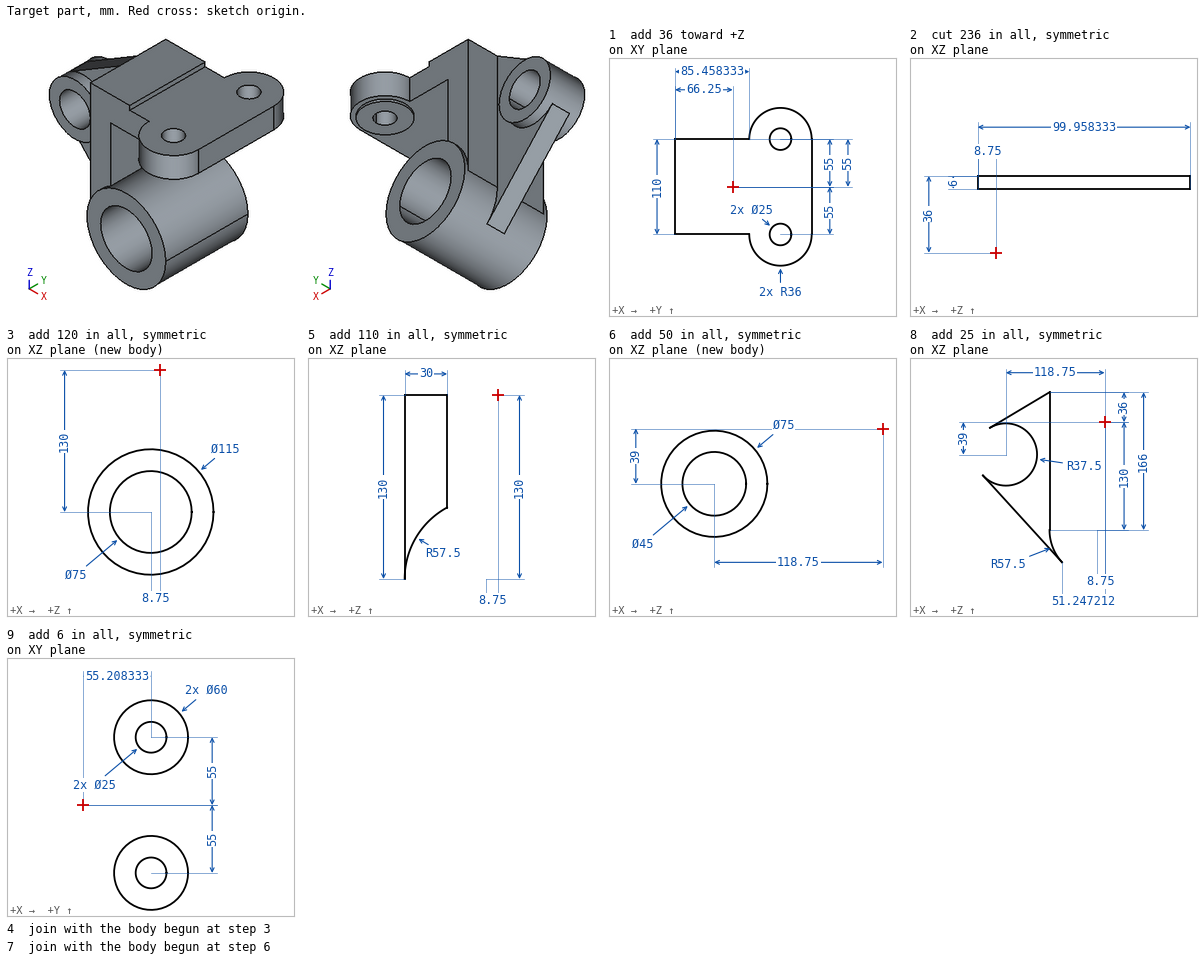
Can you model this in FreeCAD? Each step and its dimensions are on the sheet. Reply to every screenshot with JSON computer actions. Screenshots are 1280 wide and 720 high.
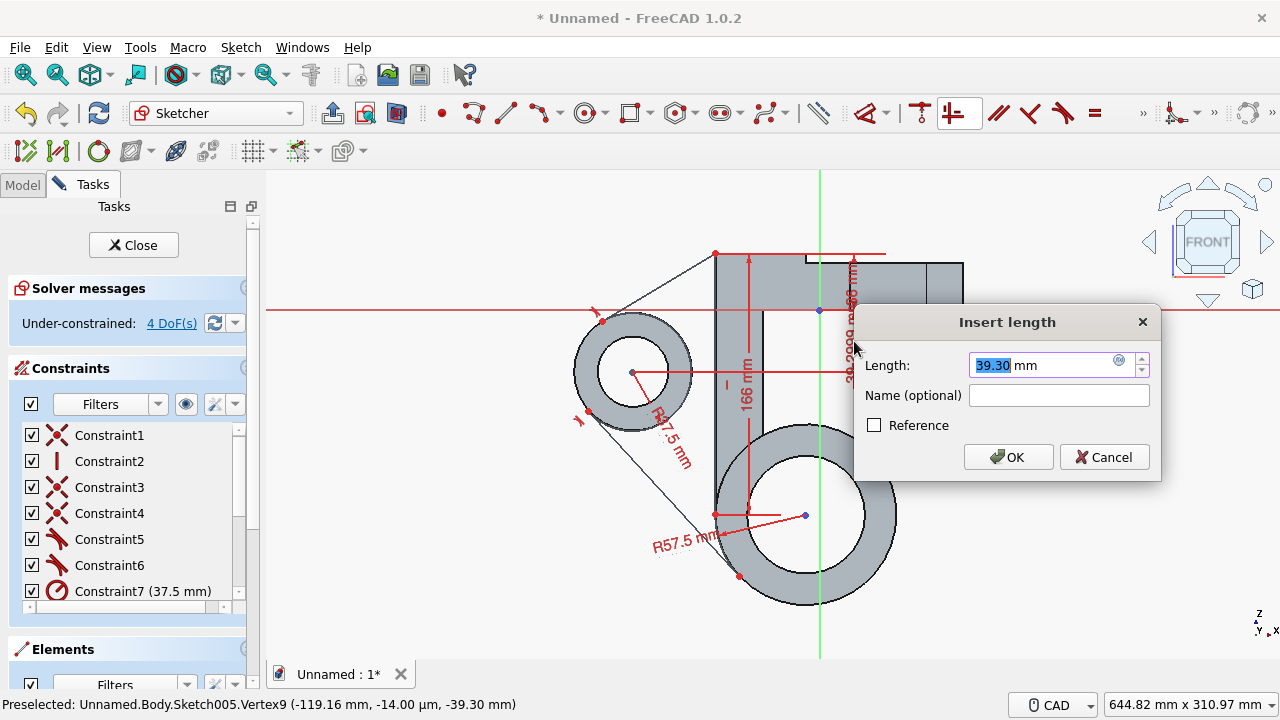
{"action": "type", "text": "39"}
{"action": "key", "text": "Return"}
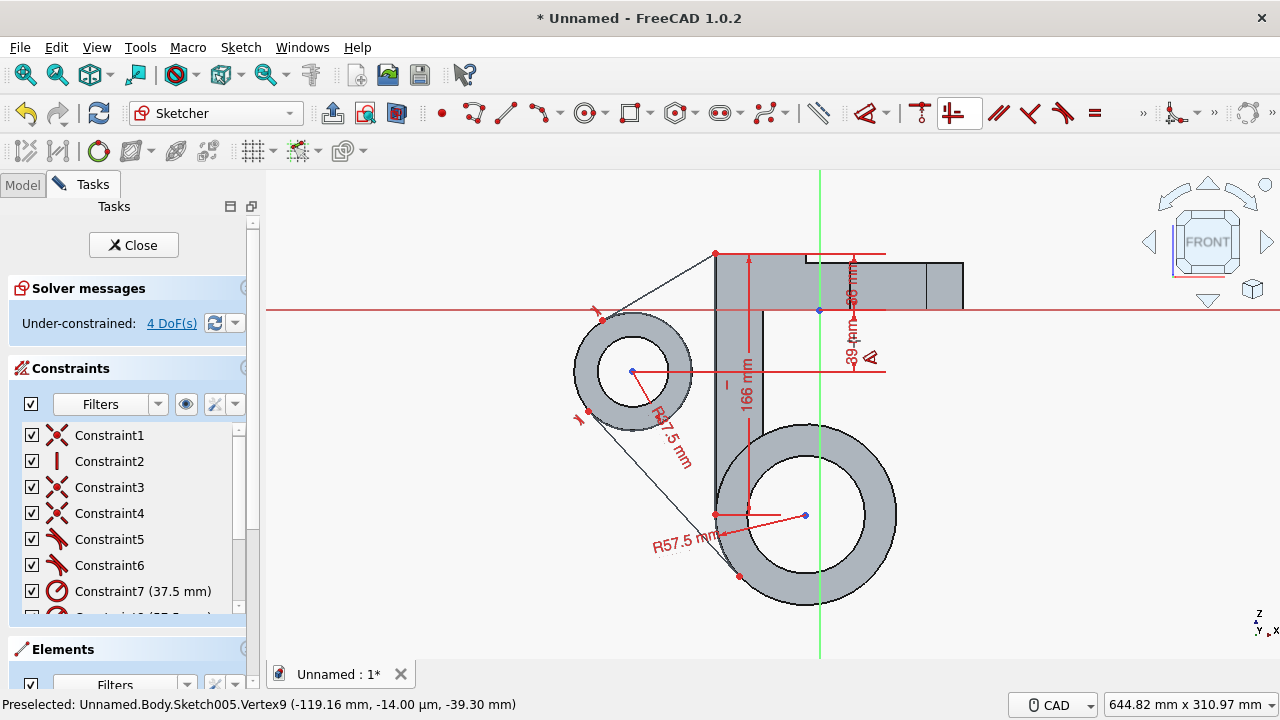
{"action": "left_click", "coordinate": [806, 515]}
{"action": "left_click", "coordinate": [854, 413]}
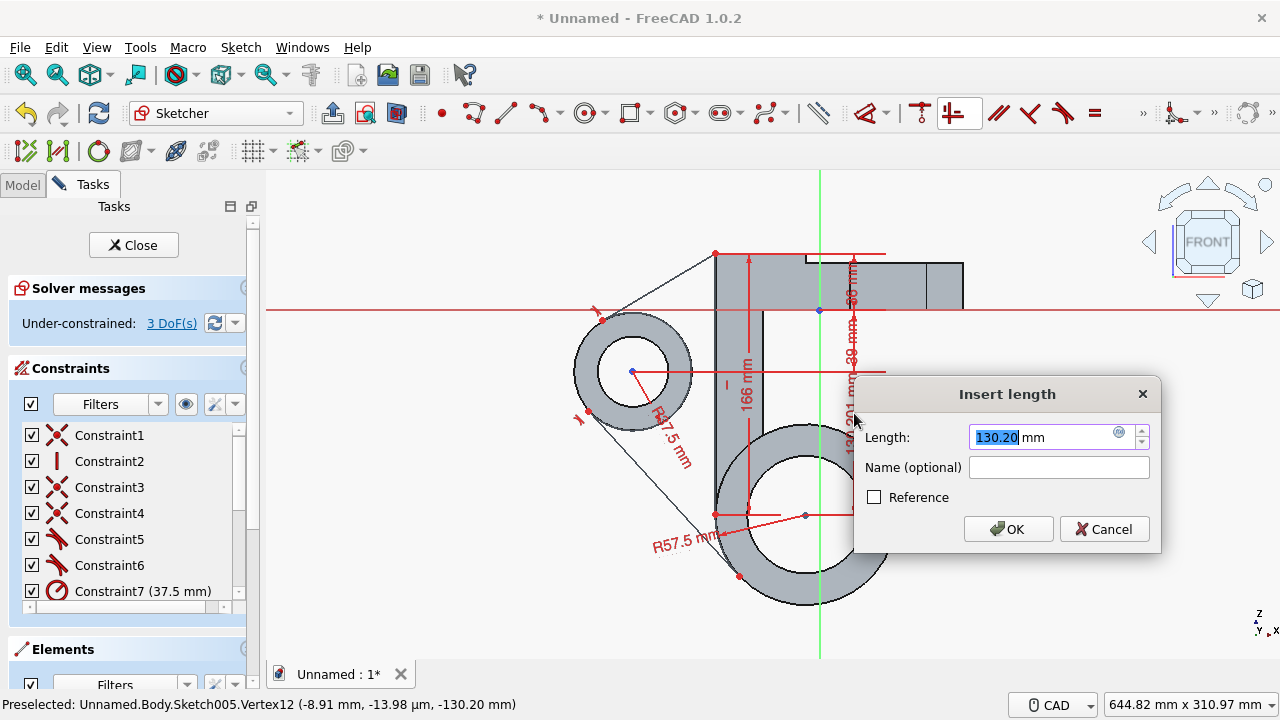
{"action": "type", "text": "130"}
{"action": "key", "text": "Return"}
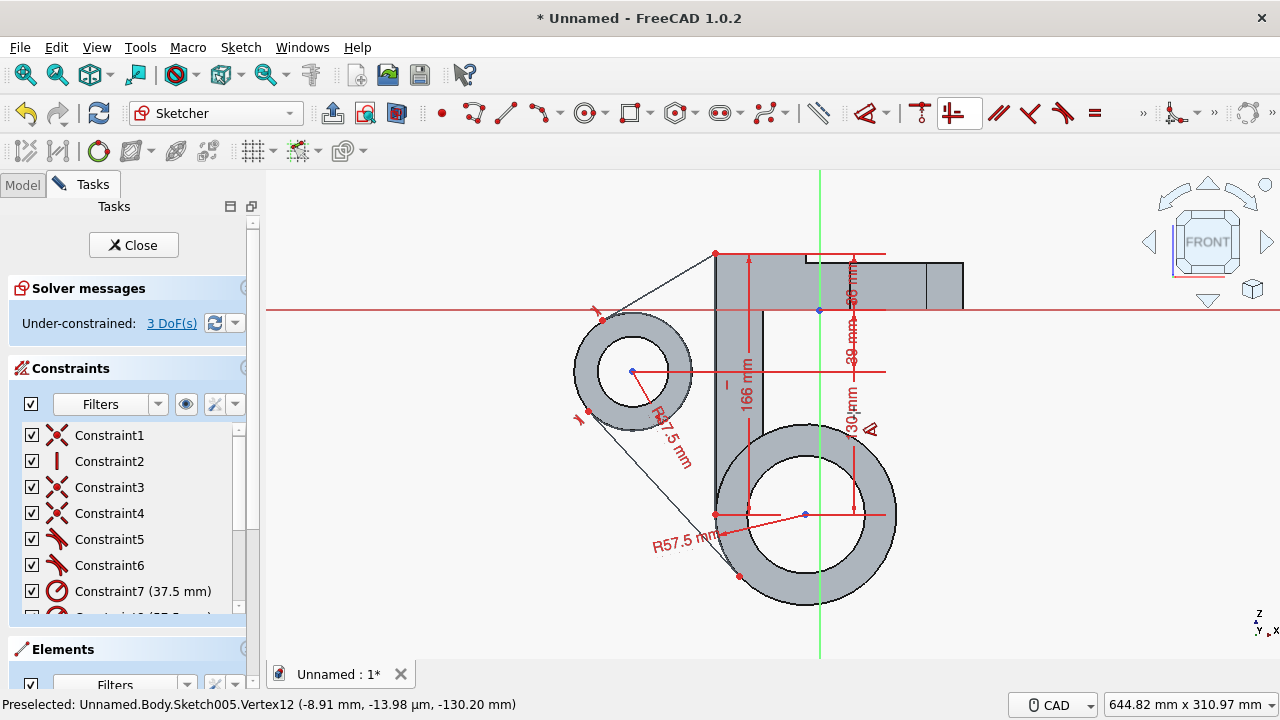
{"action": "scroll", "coordinate": [806, 515], "scroll_direction": "up", "scroll_amount": 6}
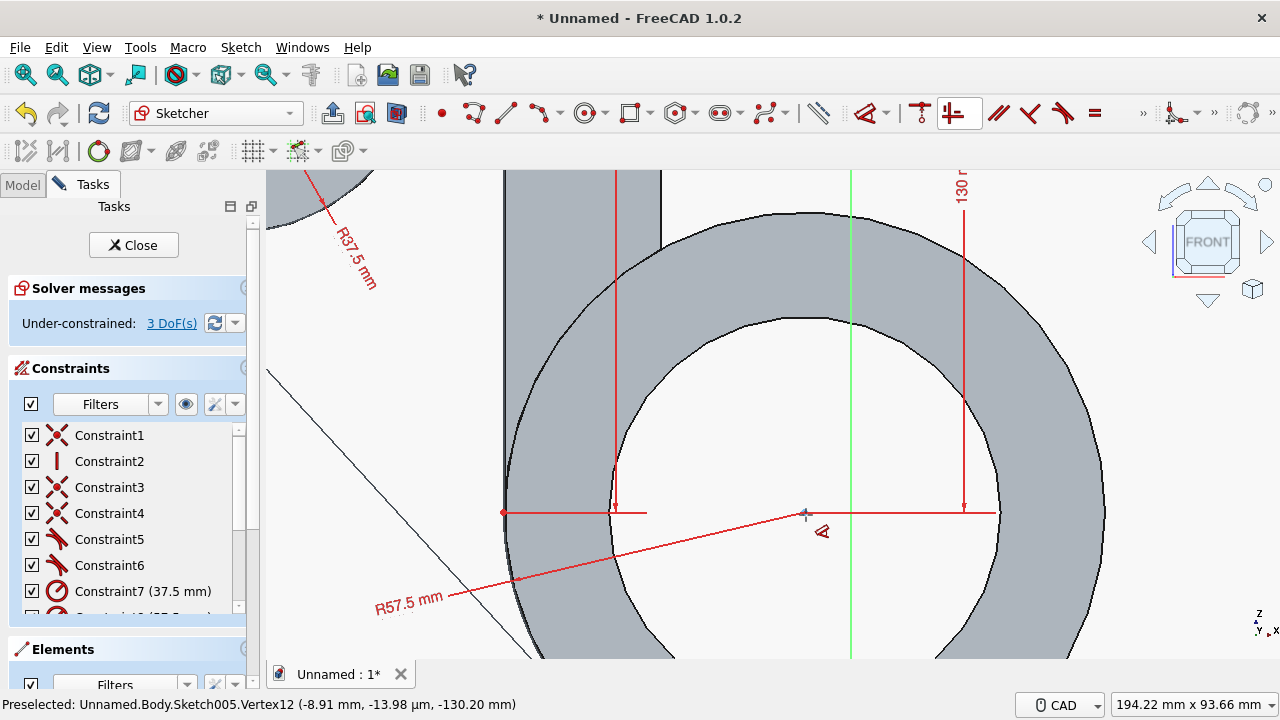
{"action": "left_click", "coordinate": [804, 513]}
{"action": "left_click", "coordinate": [827, 547]}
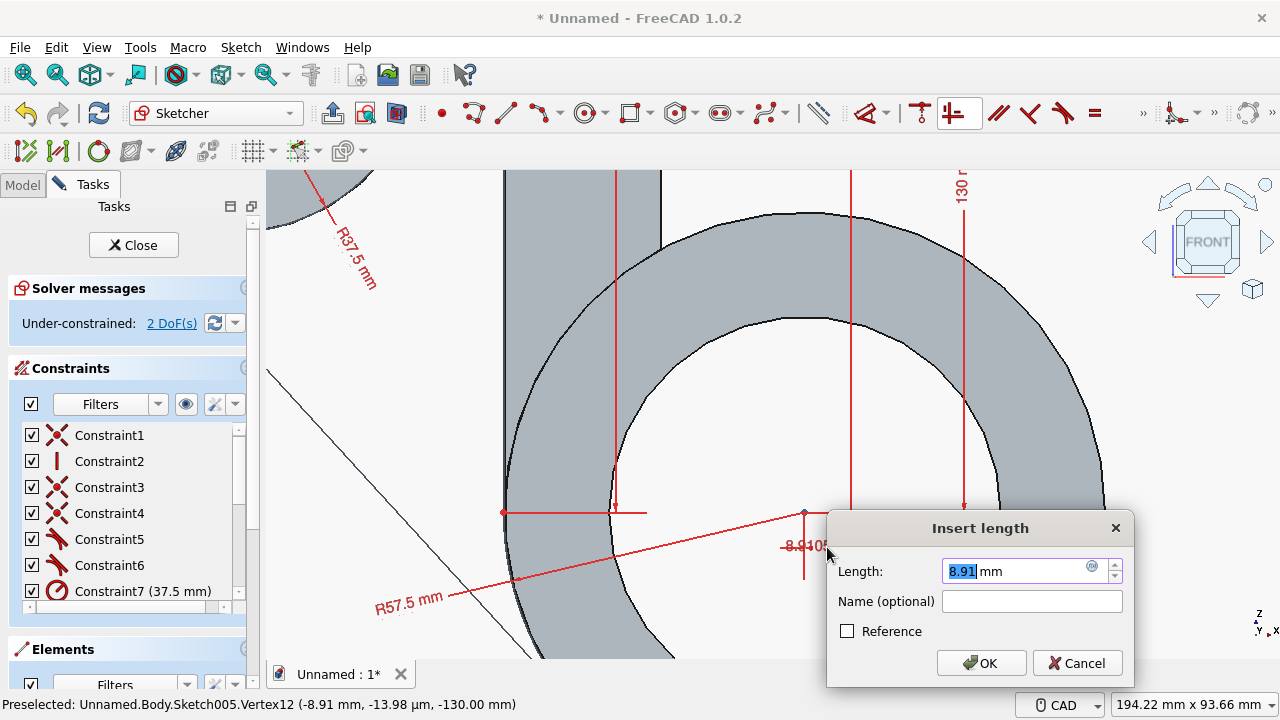
{"action": "type", "text": "8.75"}
{"action": "key", "text": "Return"}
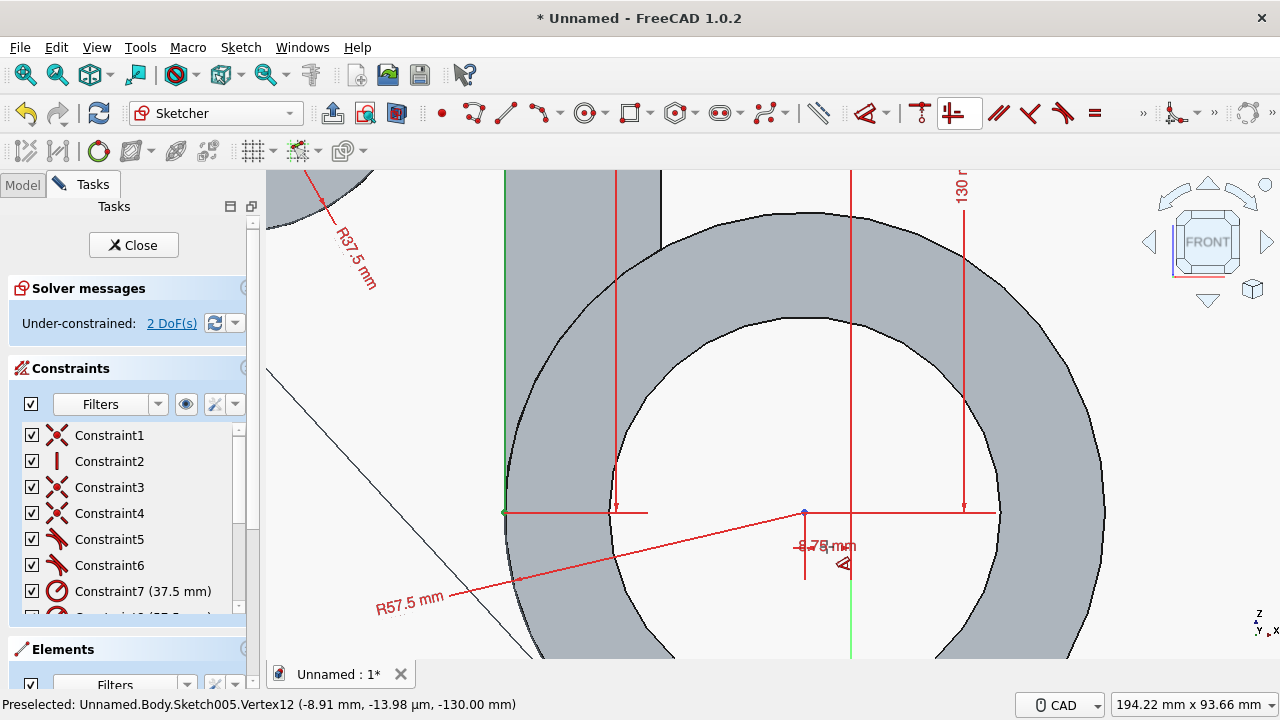
{"action": "scroll", "coordinate": [806, 515], "scroll_direction": "down", "scroll_amount": 6}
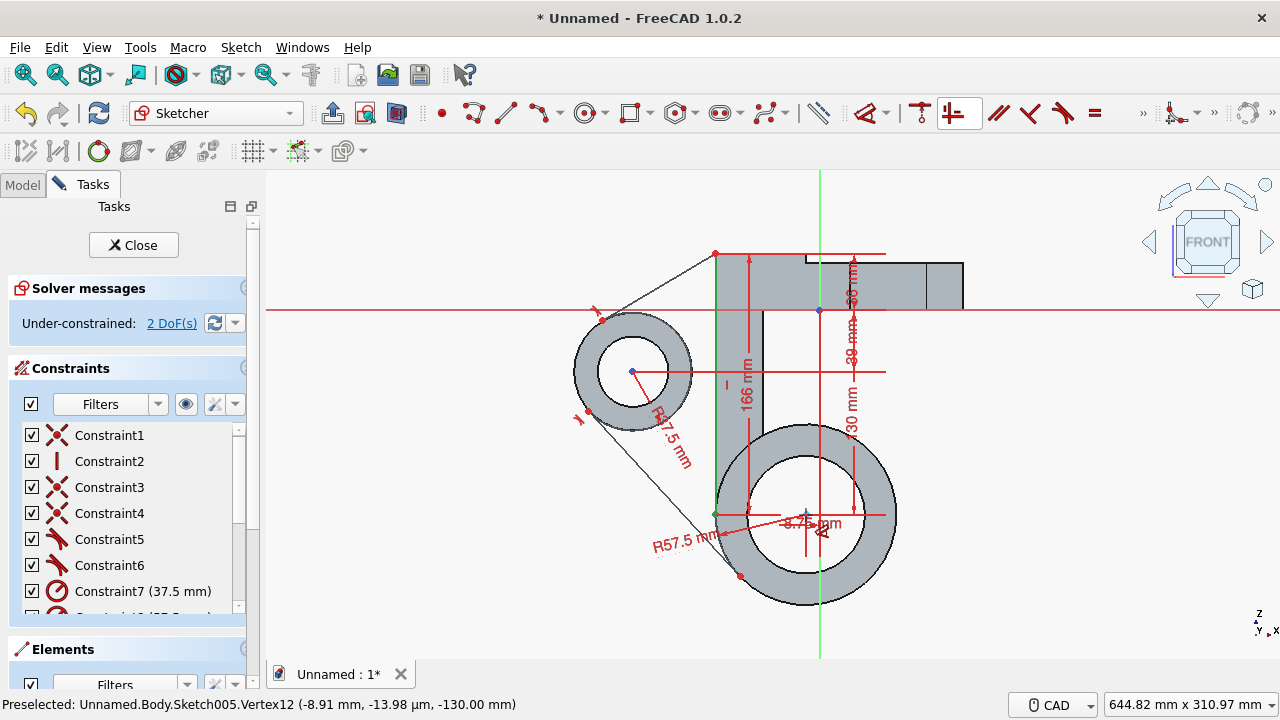
{"action": "left_click", "coordinate": [632, 372]}
{"action": "left_click", "coordinate": [769, 276]}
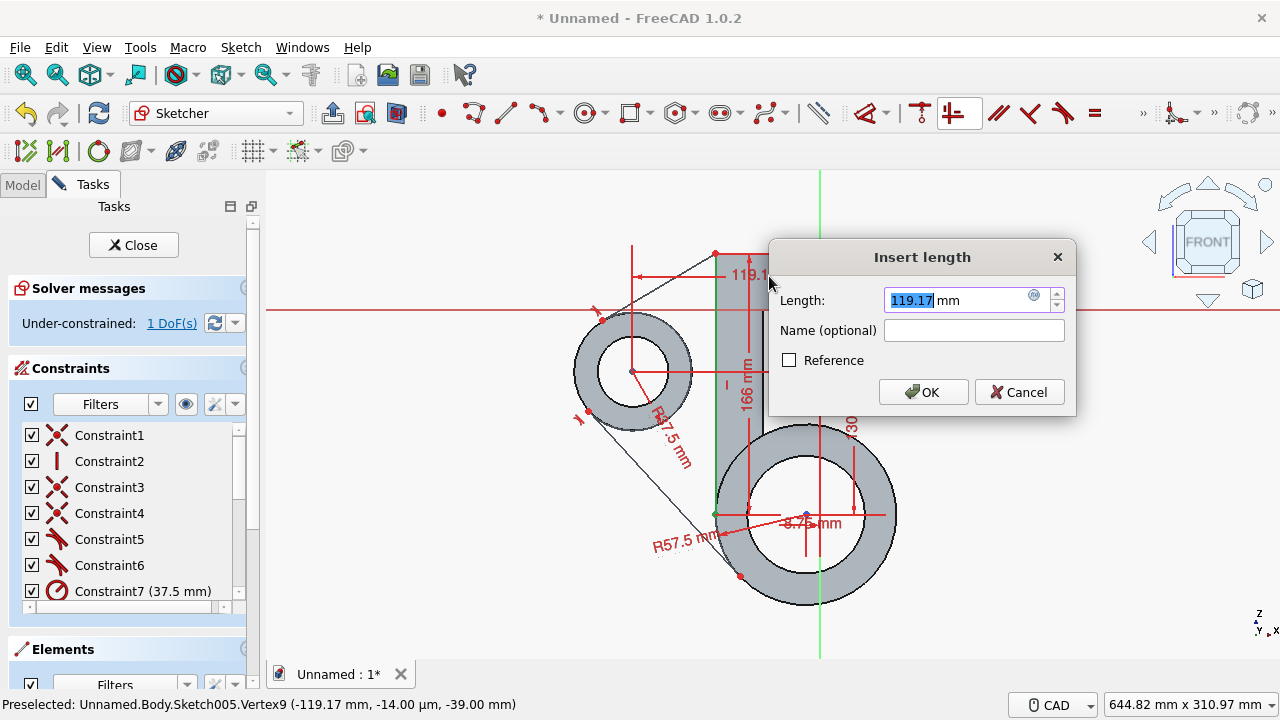
{"action": "type", "text": "118.75"}
{"action": "key", "text": "Return"}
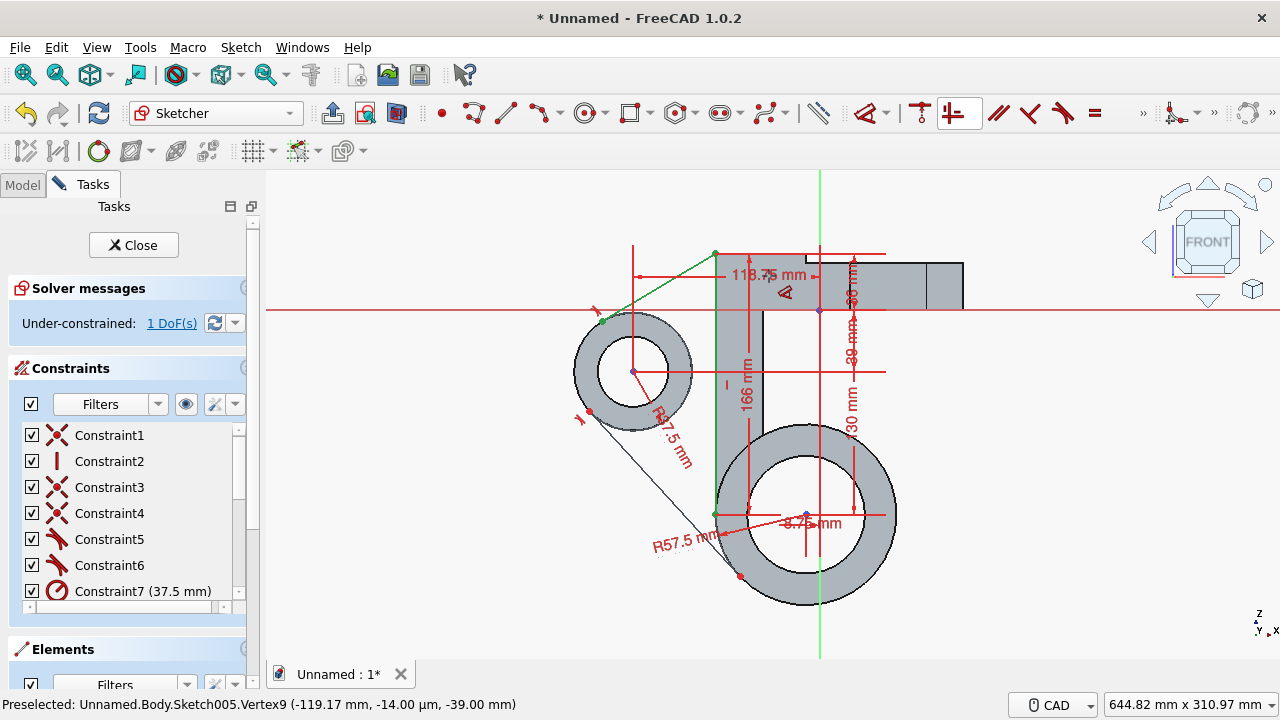
{"action": "left_click", "coordinate": [740, 577]}
{"action": "left_click", "coordinate": [780, 611]}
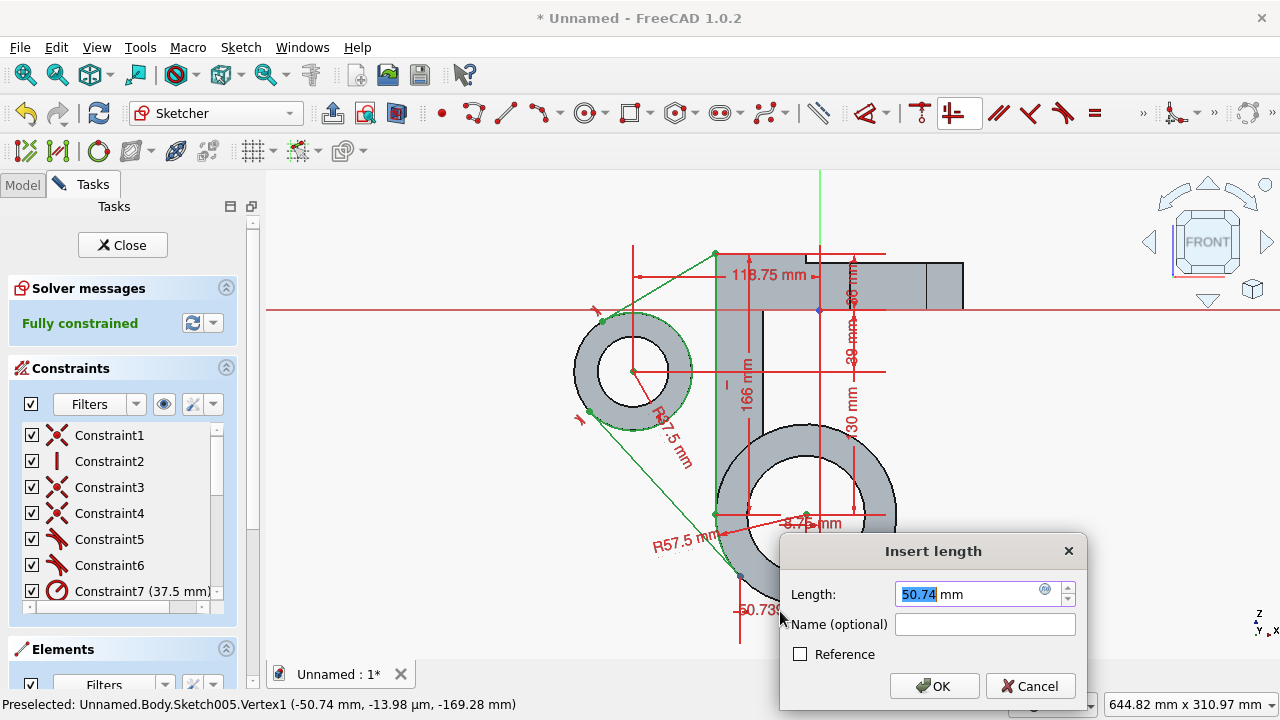
{"action": "type", "text": "51.247212"}
{"action": "key", "text": "Return"}
{"action": "key", "text": "Escape"}